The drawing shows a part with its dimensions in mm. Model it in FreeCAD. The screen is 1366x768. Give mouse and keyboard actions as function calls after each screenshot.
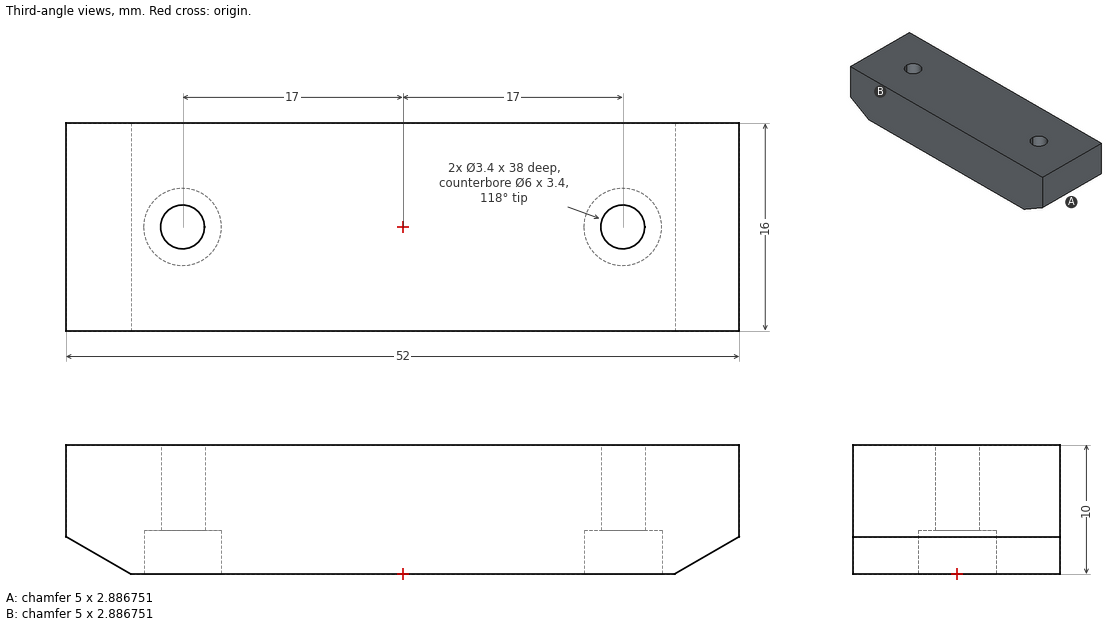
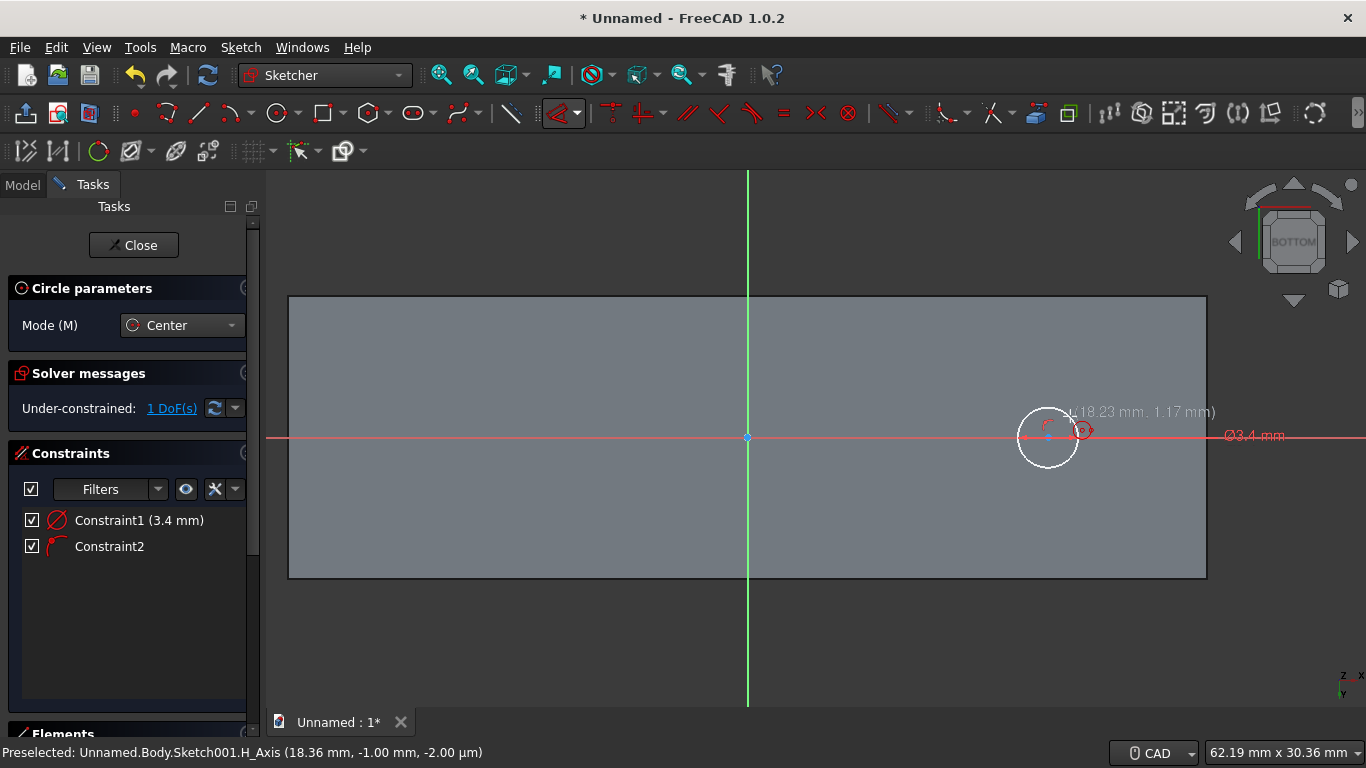
click(447, 438)
move(468, 416)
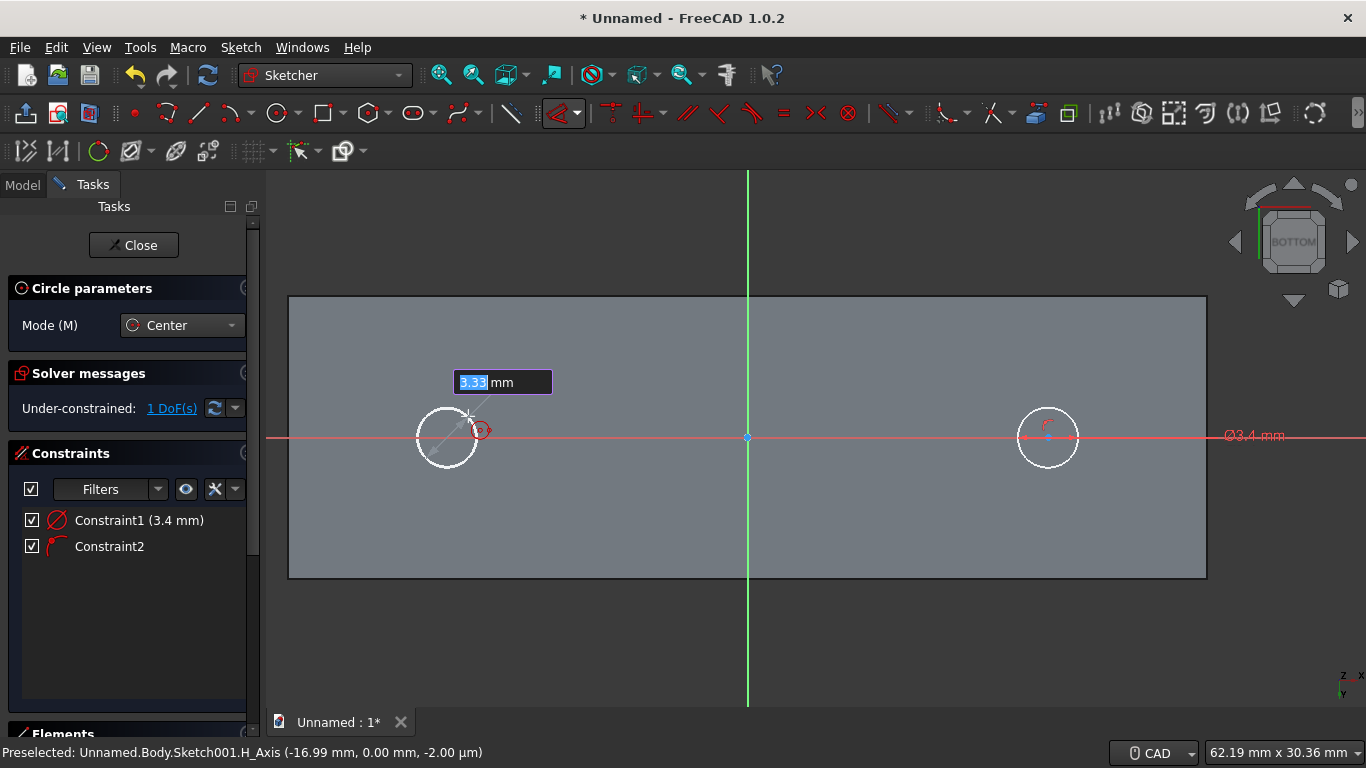
text(3.4)
key(Return)
key(Escape)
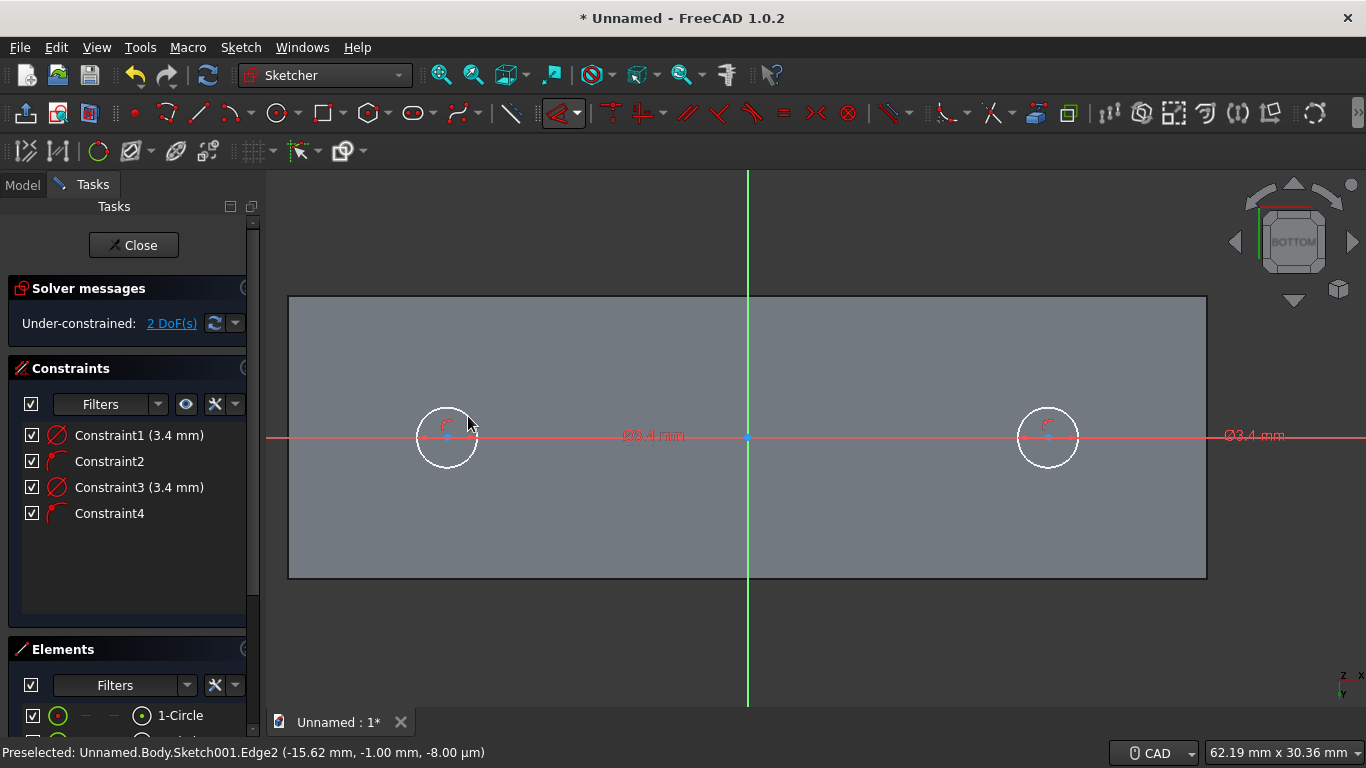
click(558, 114)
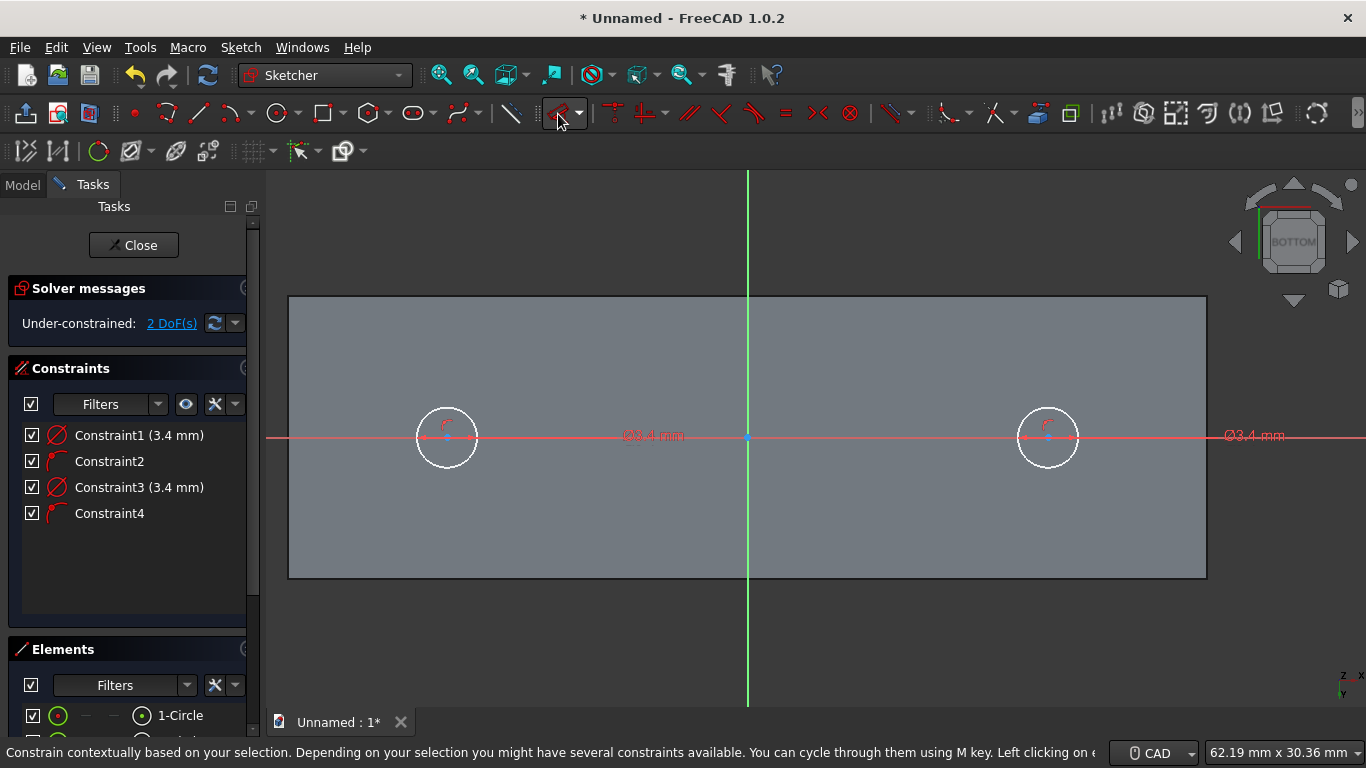
click(1048, 438)
click(898, 472)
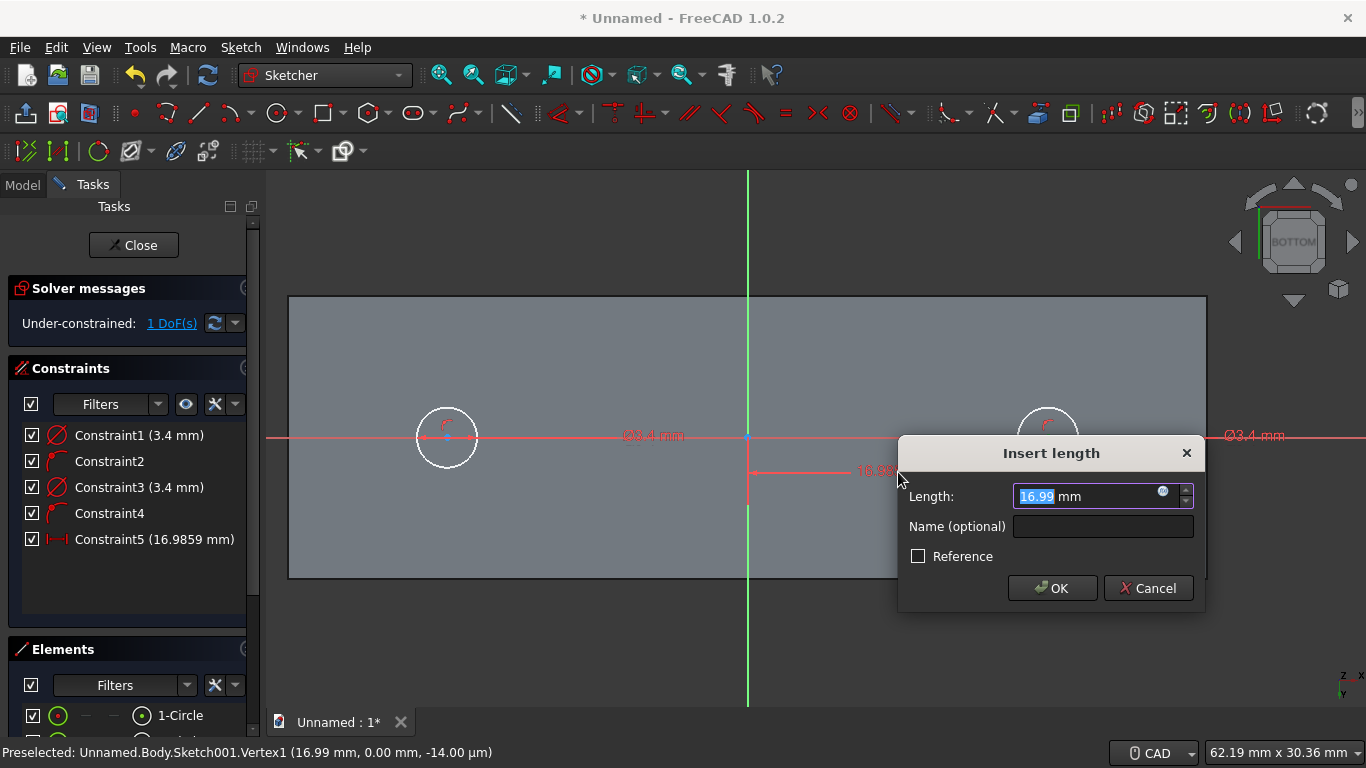
text(17)
key(Return)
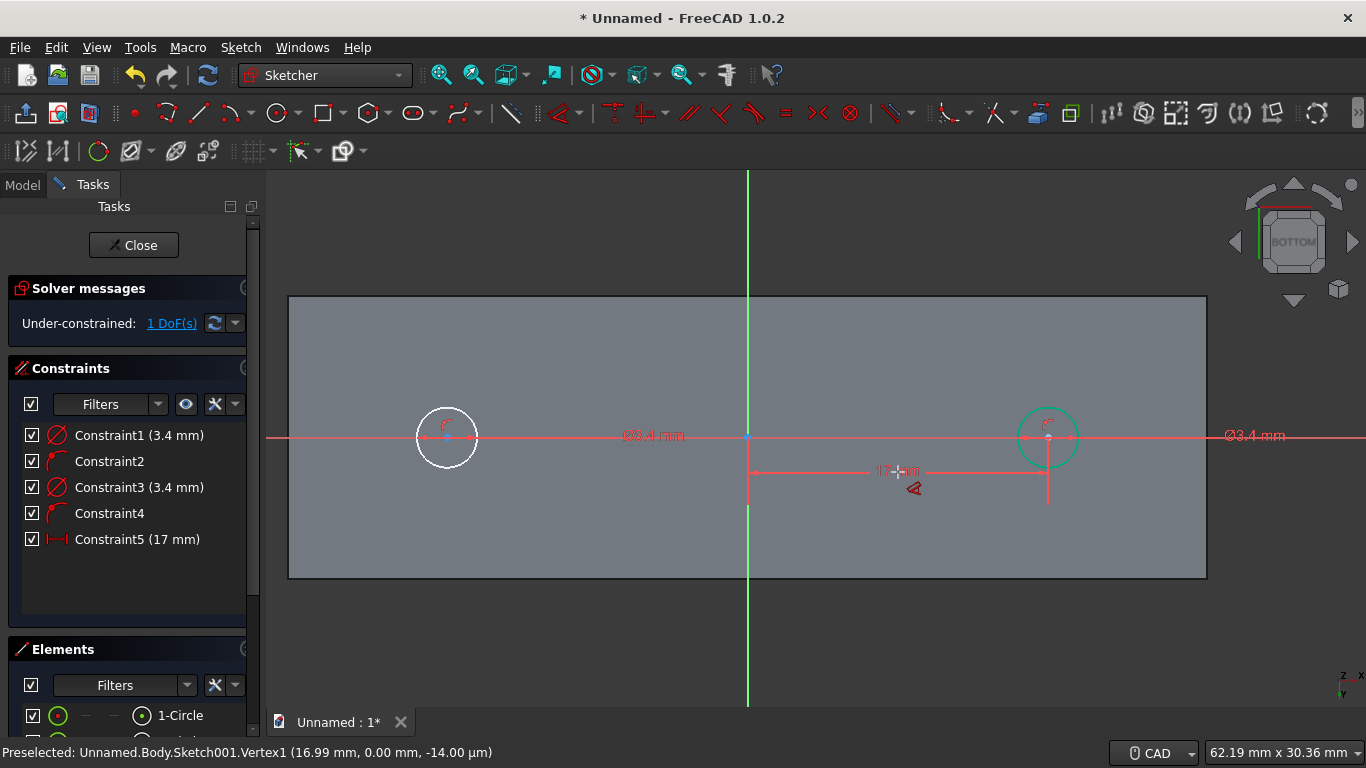
click(447, 438)
click(597, 472)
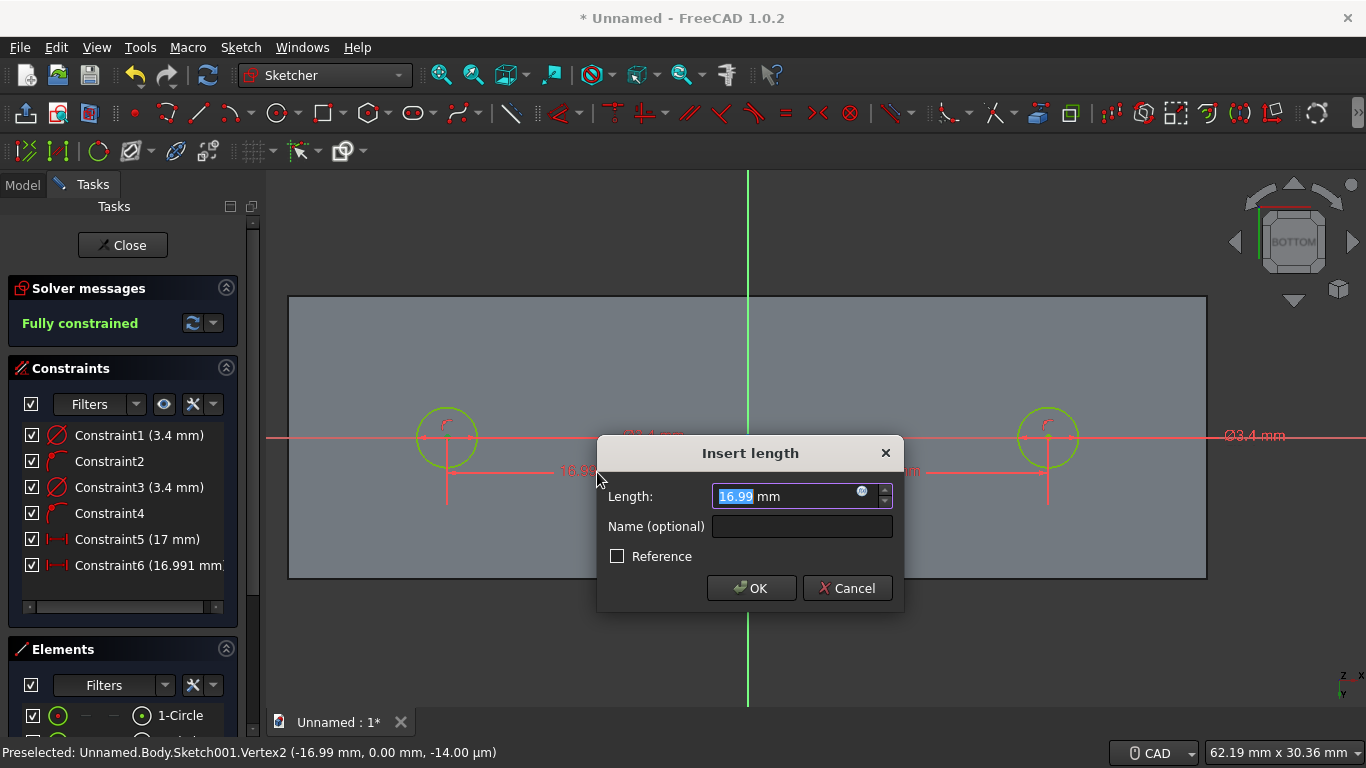
text(17)
key(Return)
key(Escape)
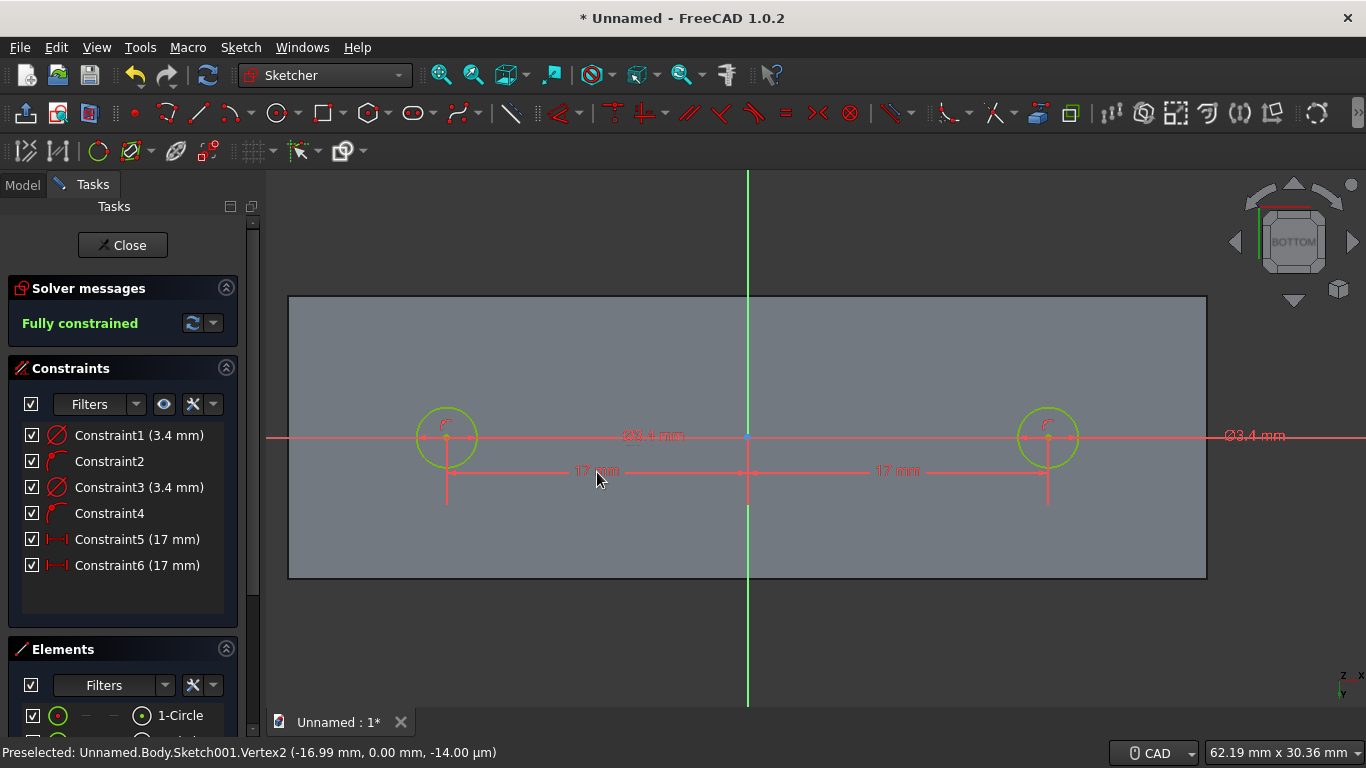
click(123, 245)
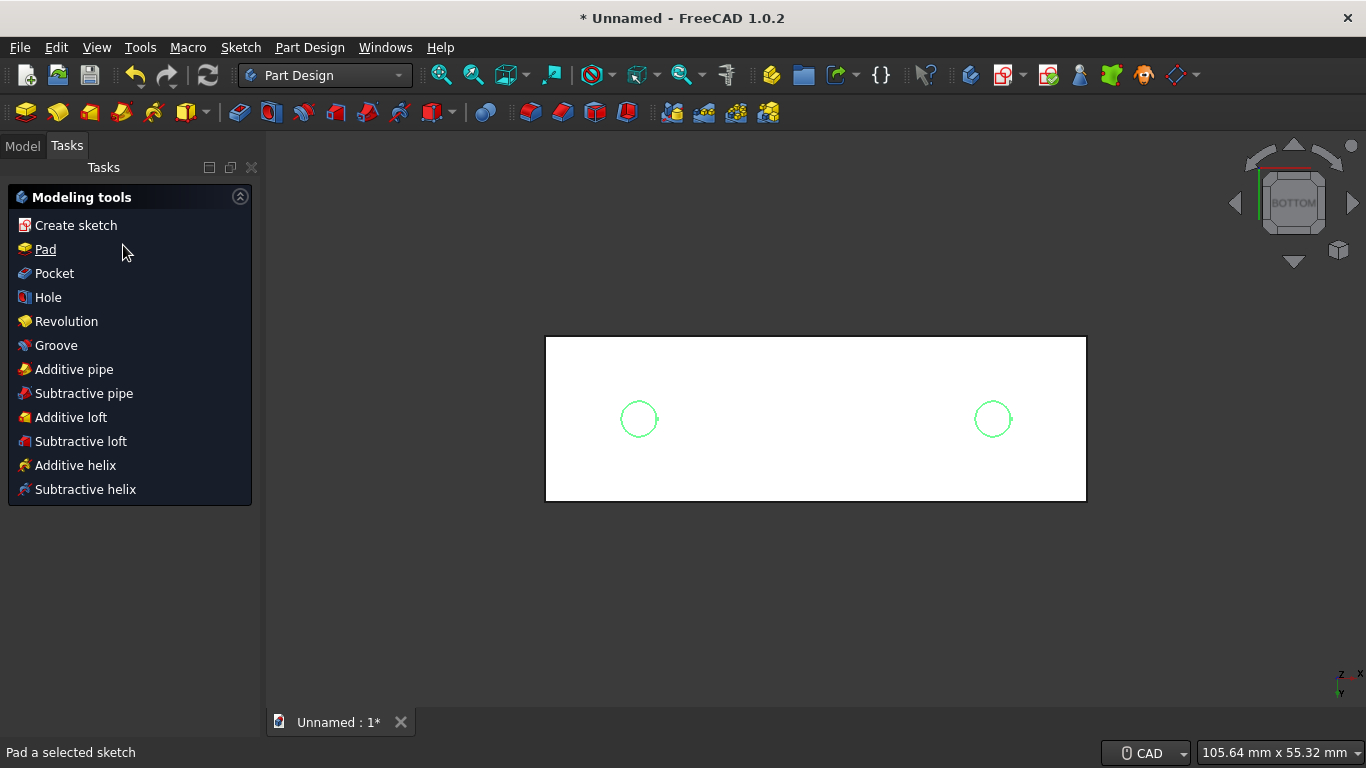
click(272, 112)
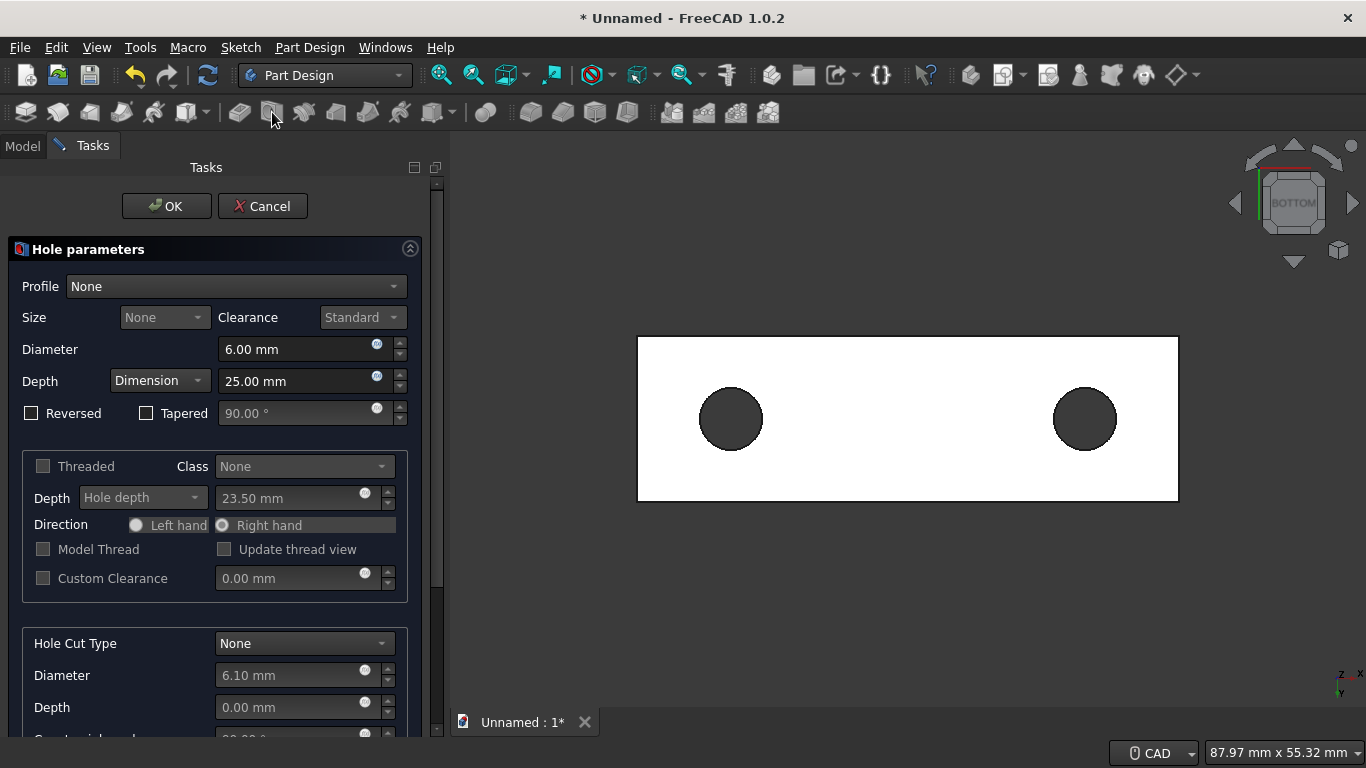
triple_click(305, 349)